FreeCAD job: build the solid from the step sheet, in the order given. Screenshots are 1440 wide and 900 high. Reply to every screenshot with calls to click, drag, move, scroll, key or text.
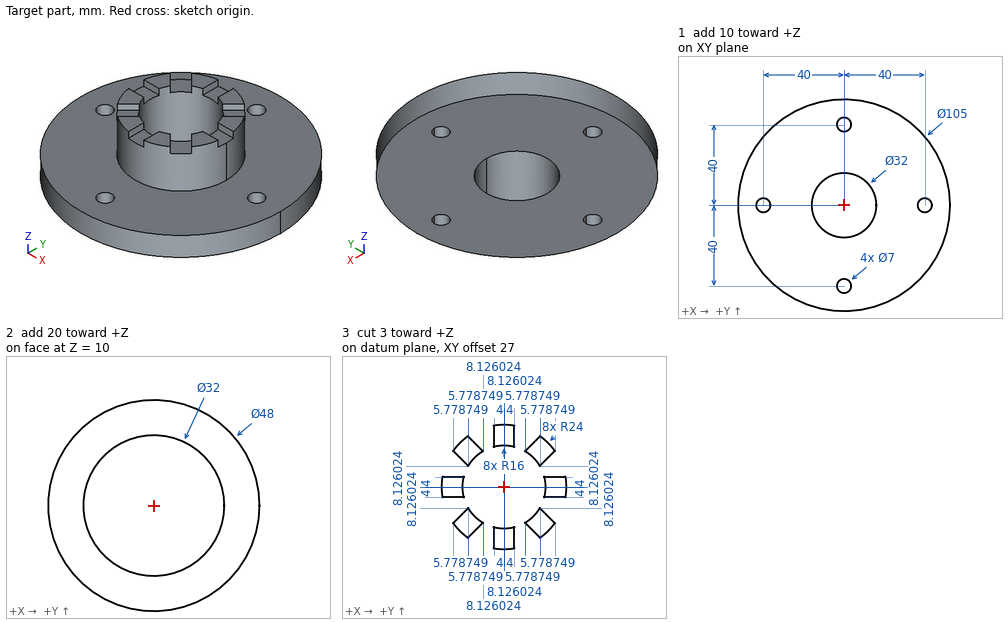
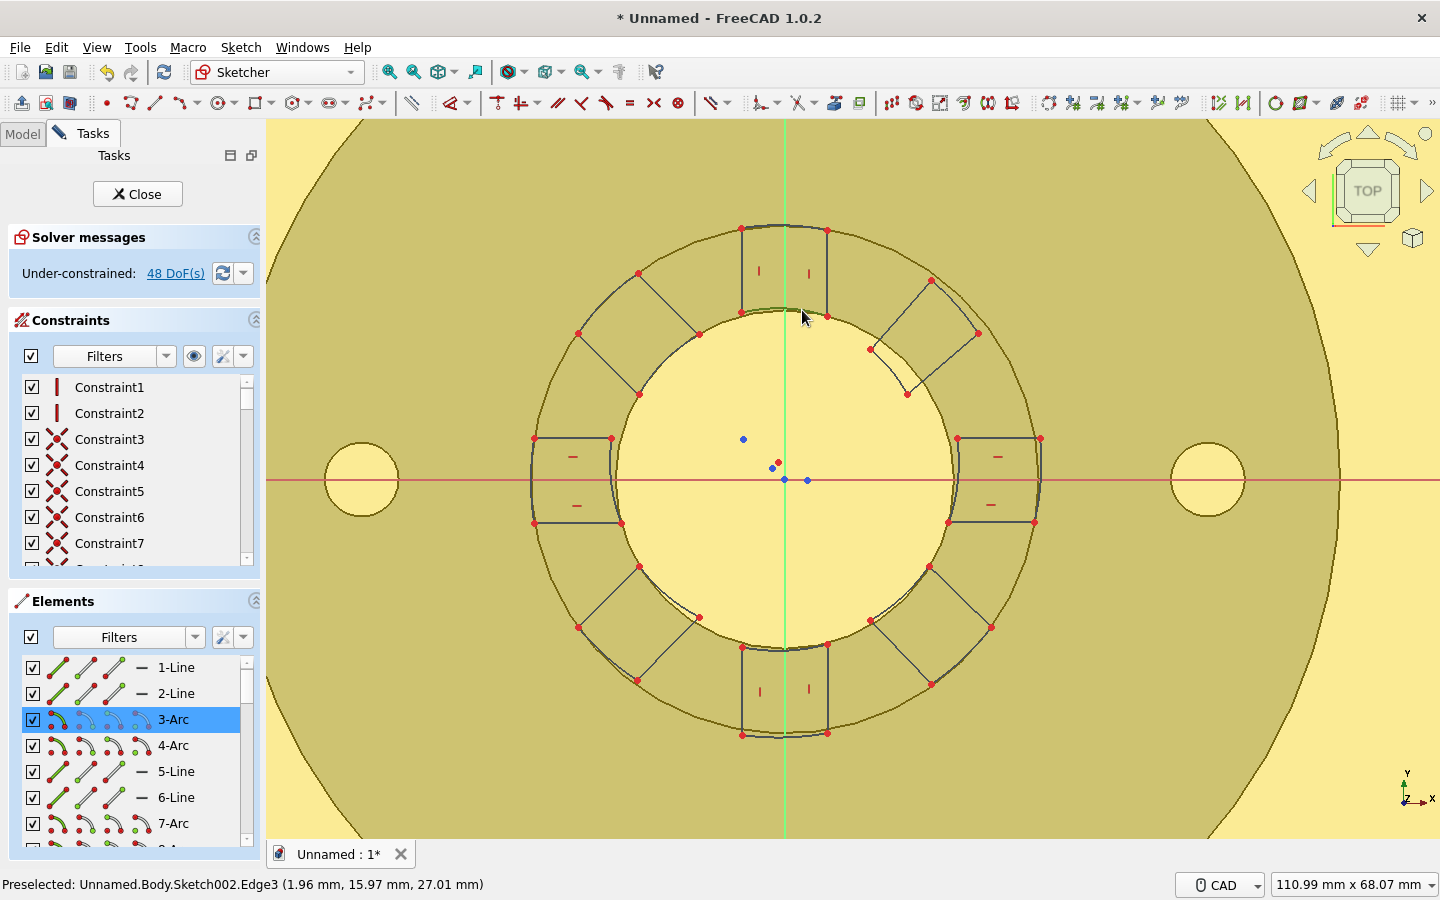
click(532, 464)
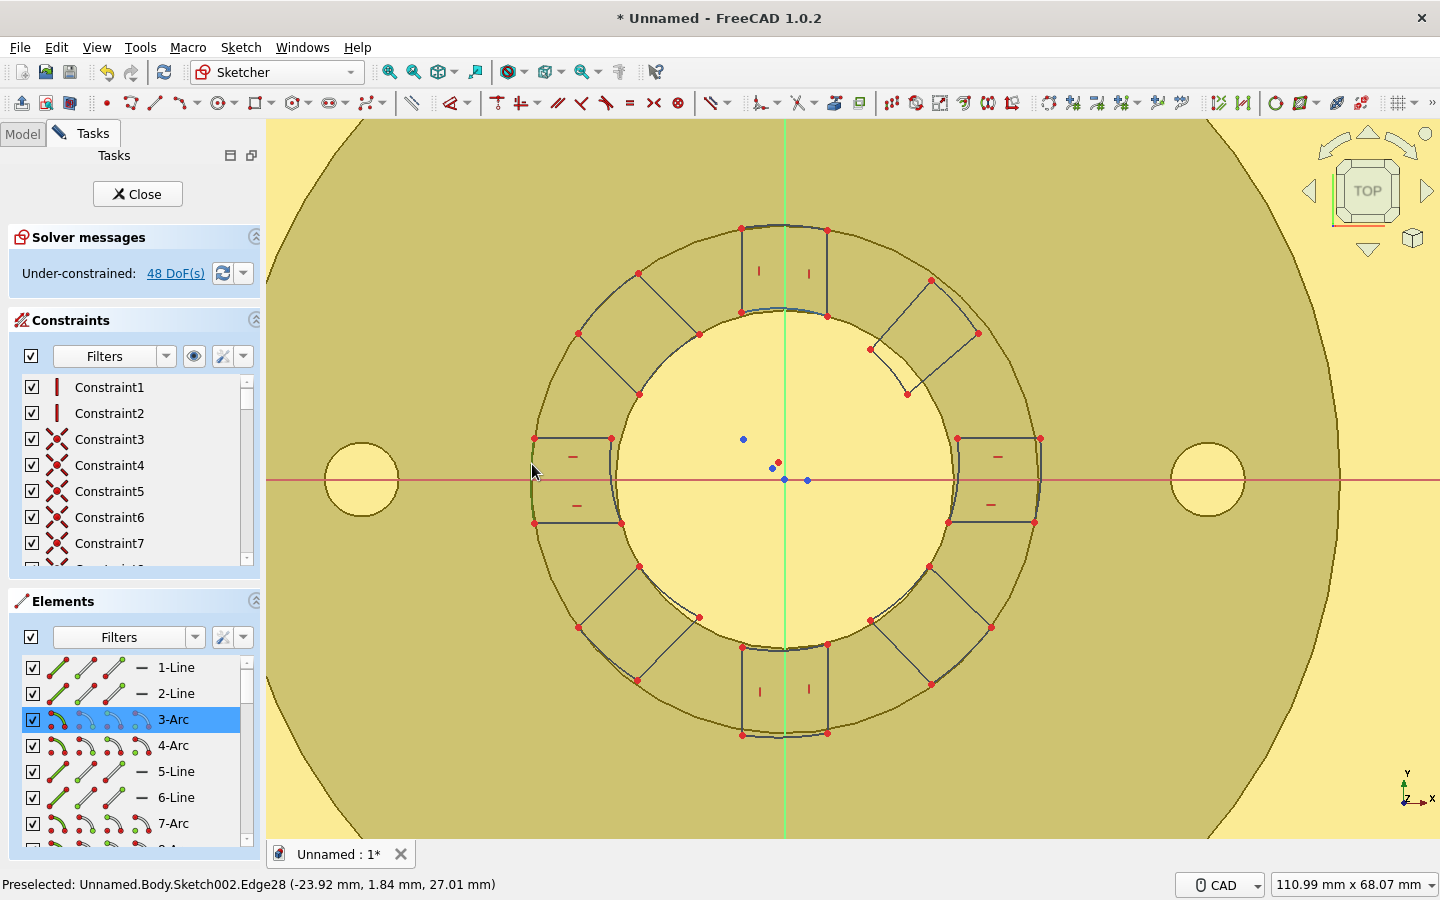
click(498, 104)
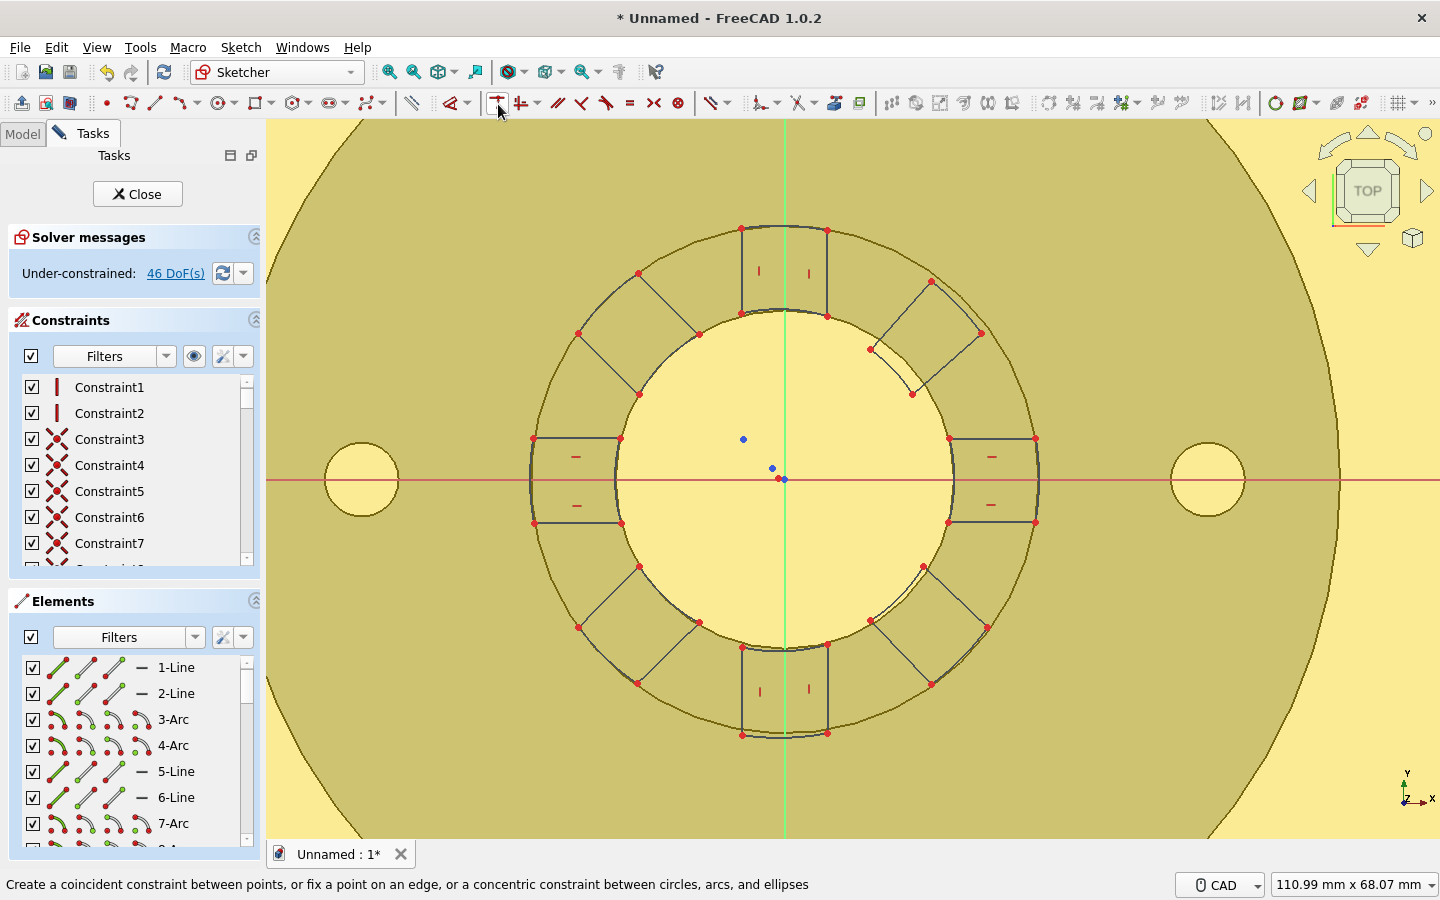
click(802, 311)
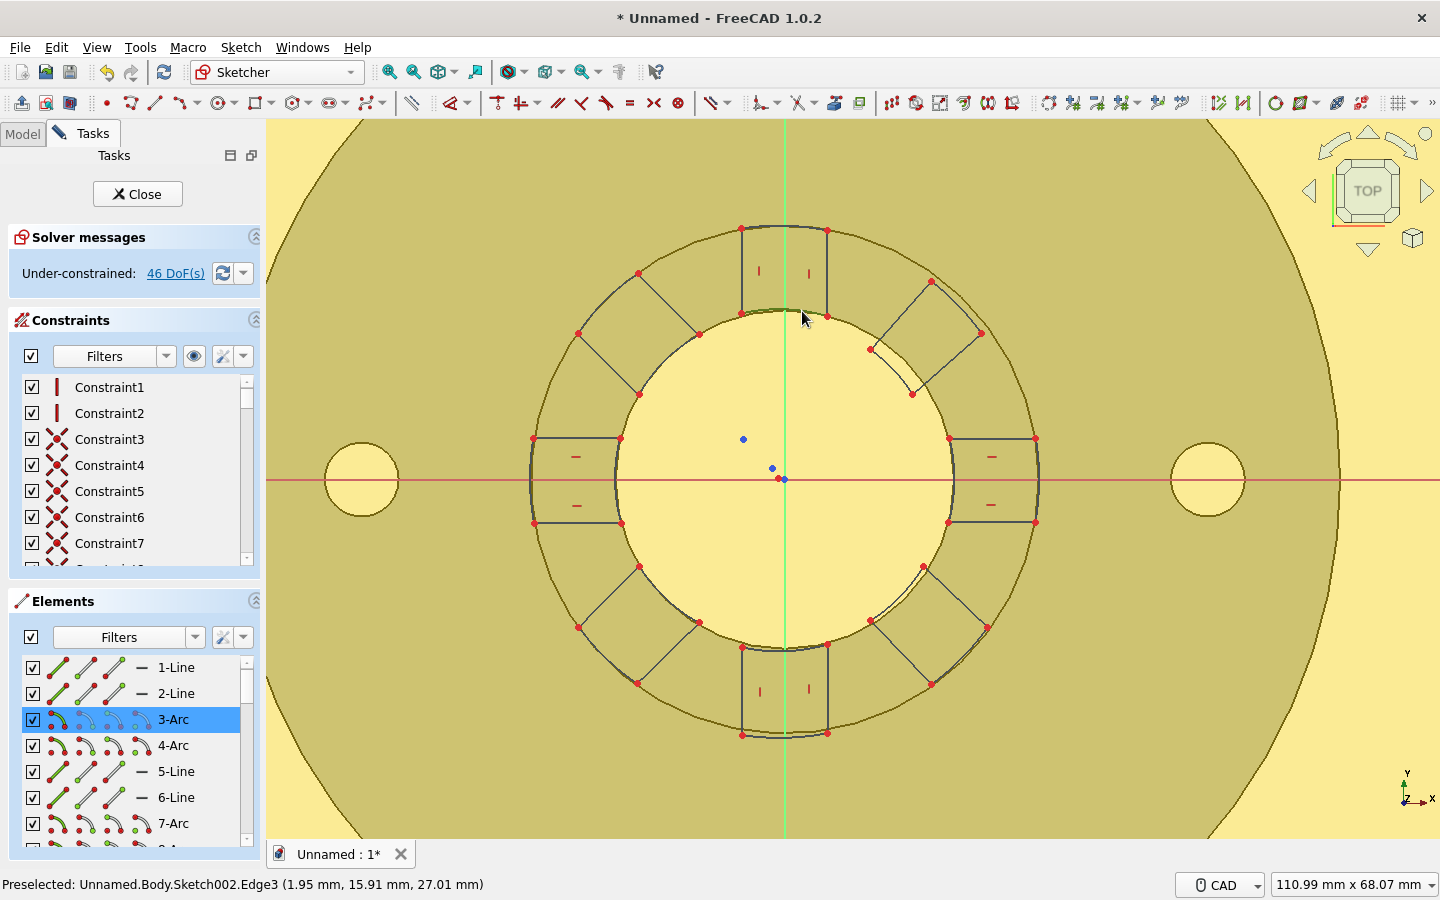
click(678, 349)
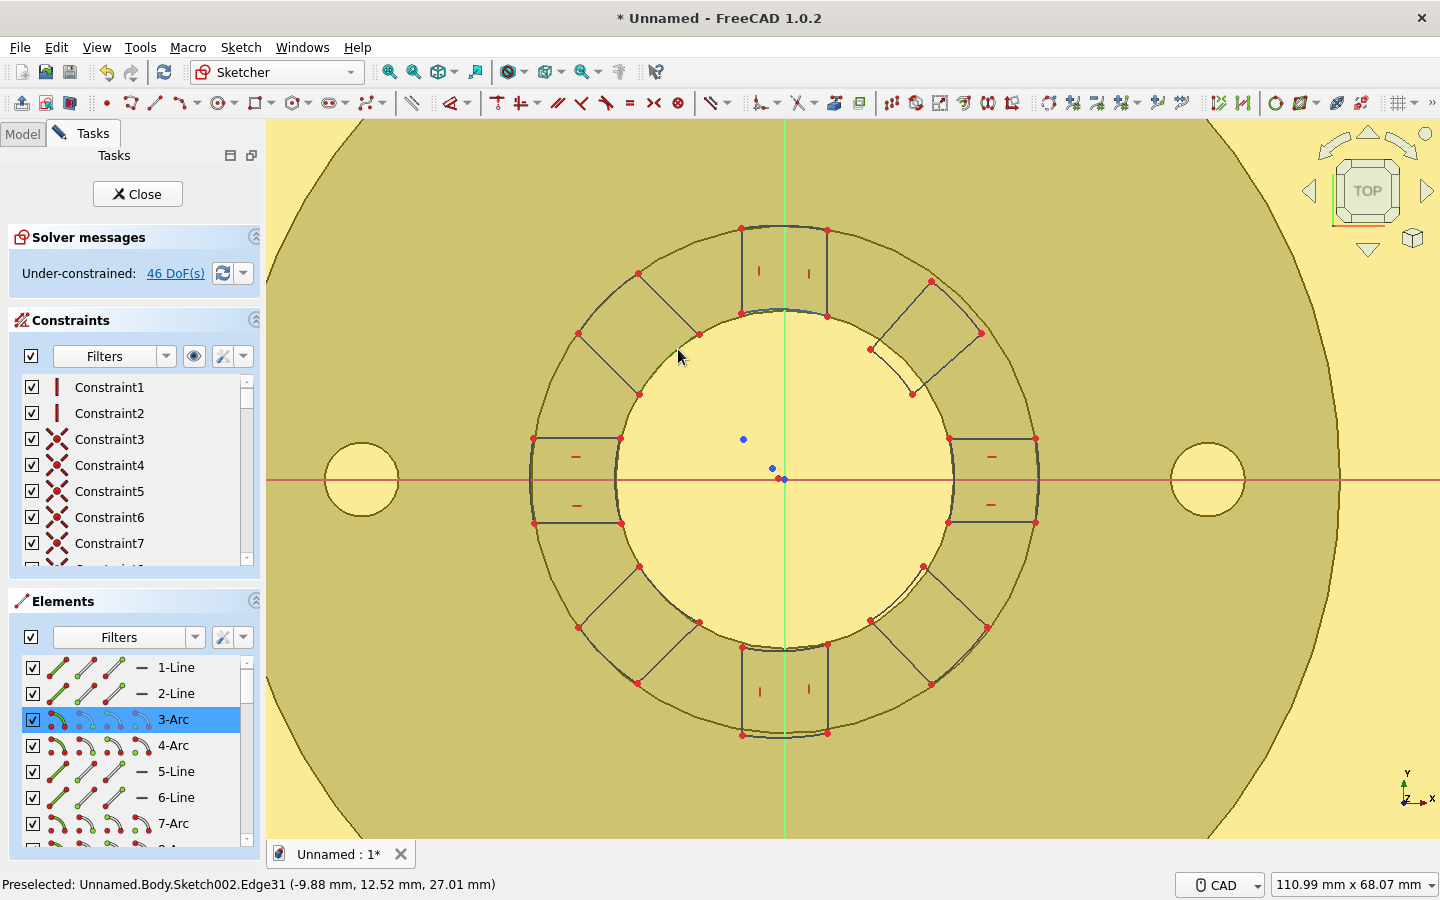
click(498, 104)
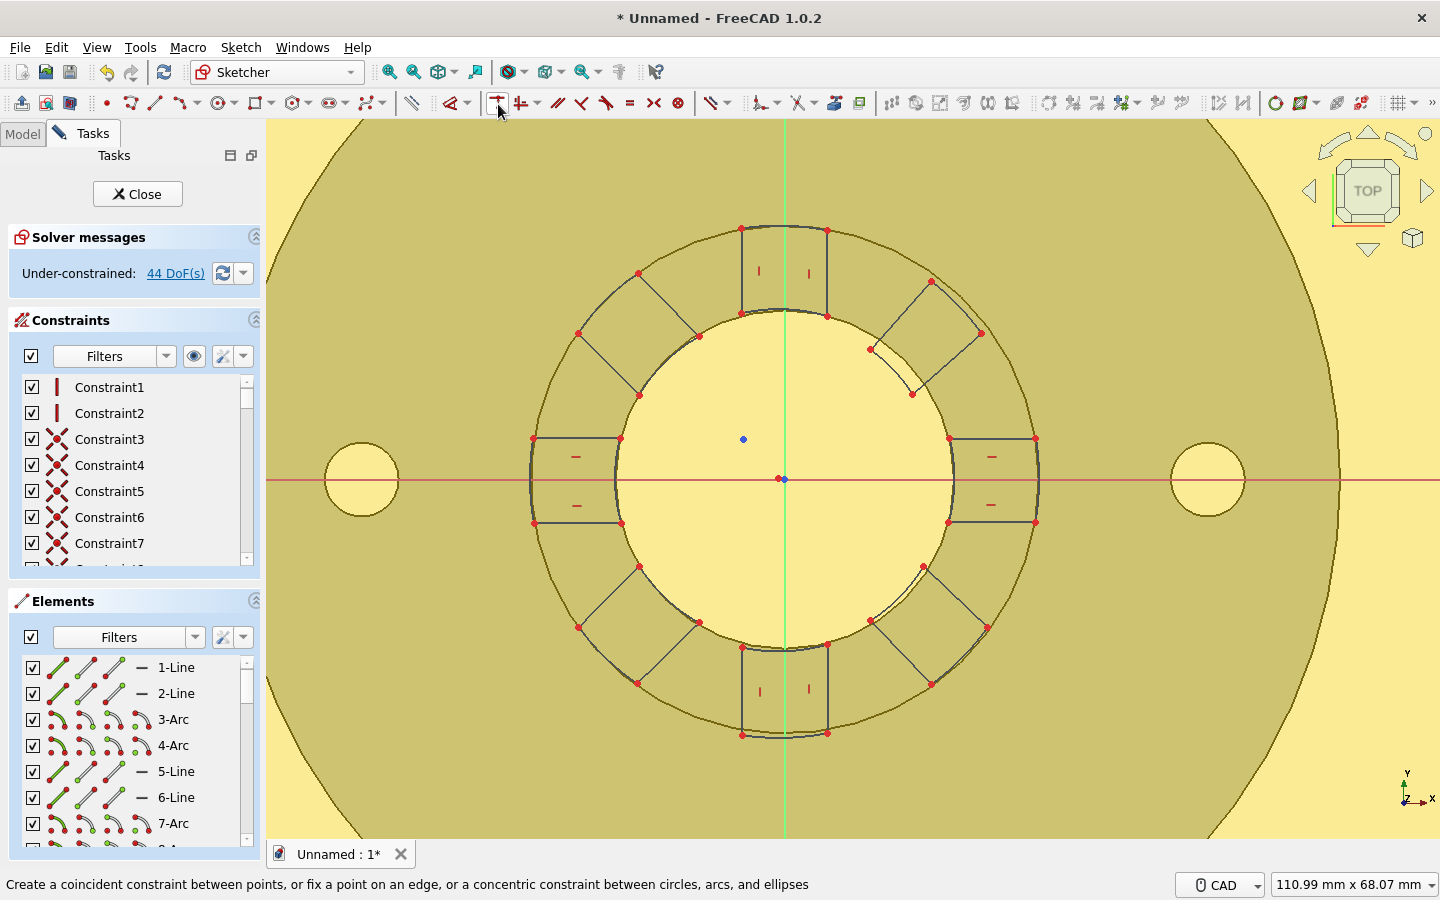
click(802, 311)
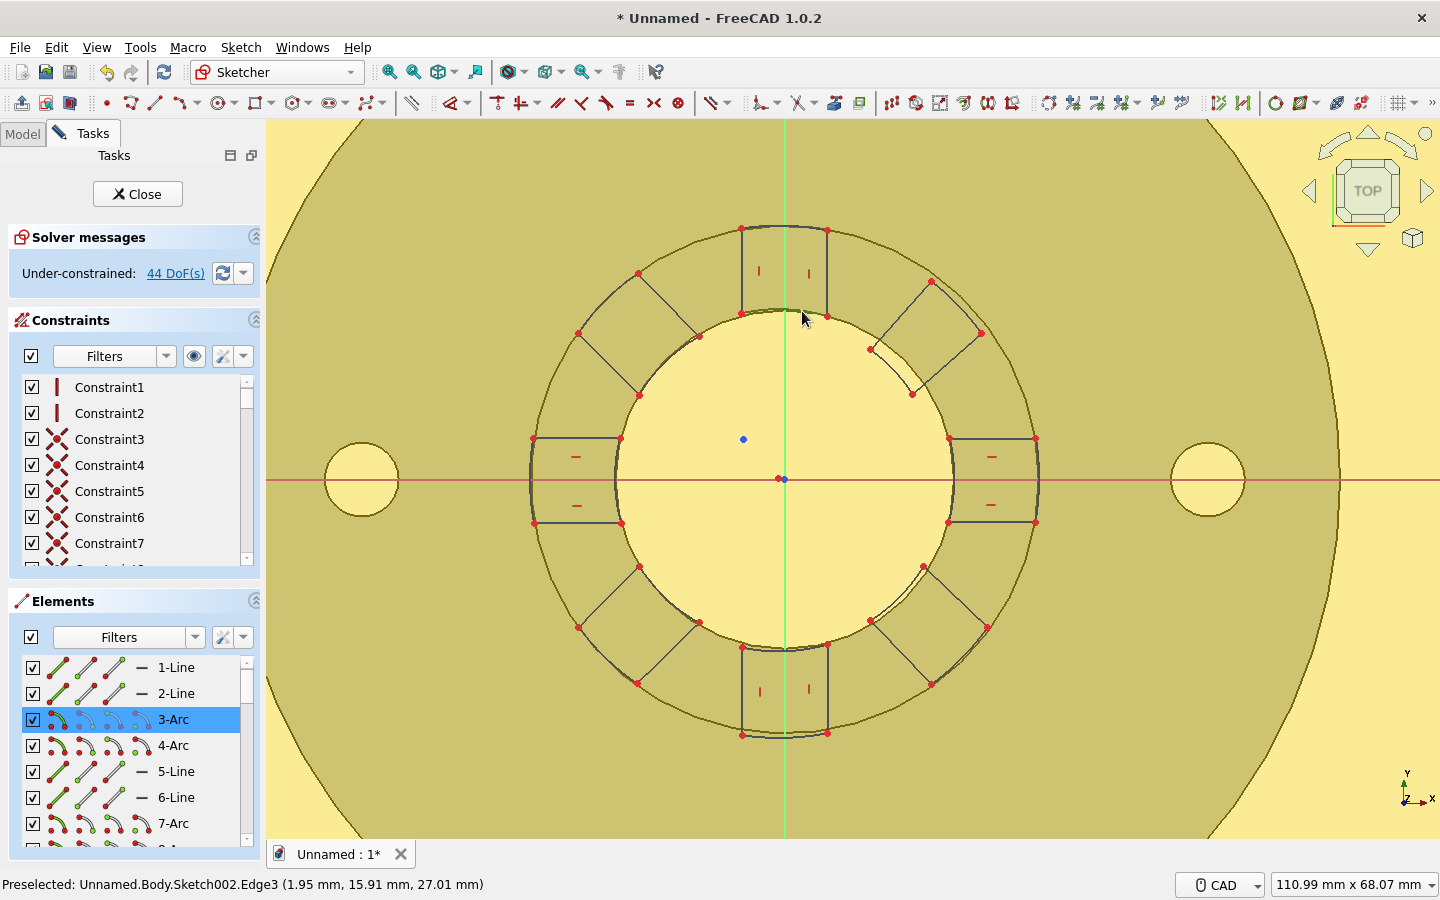
click(617, 289)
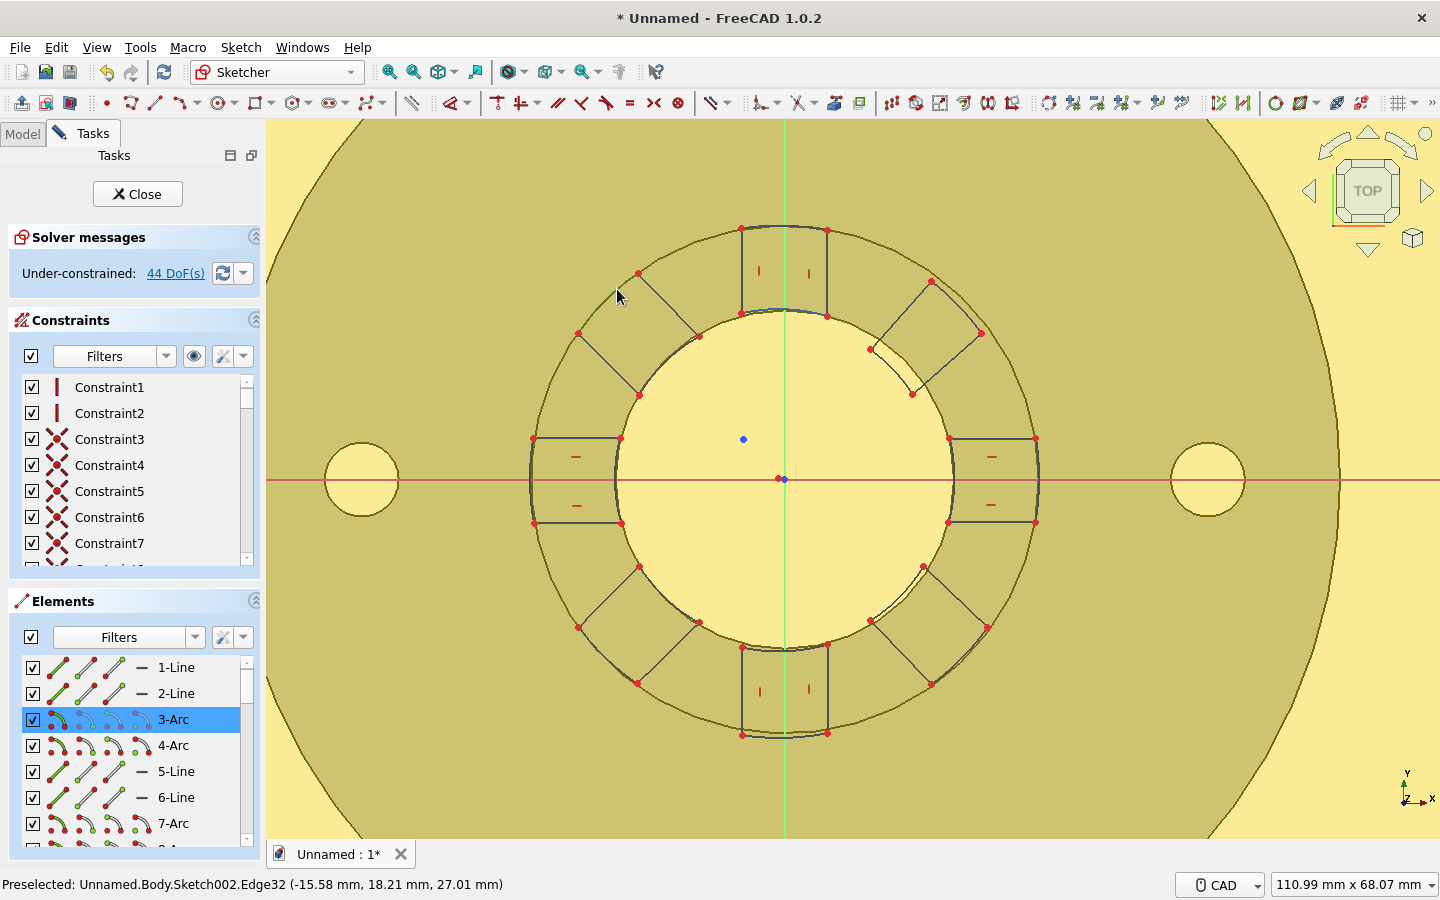
click(498, 104)